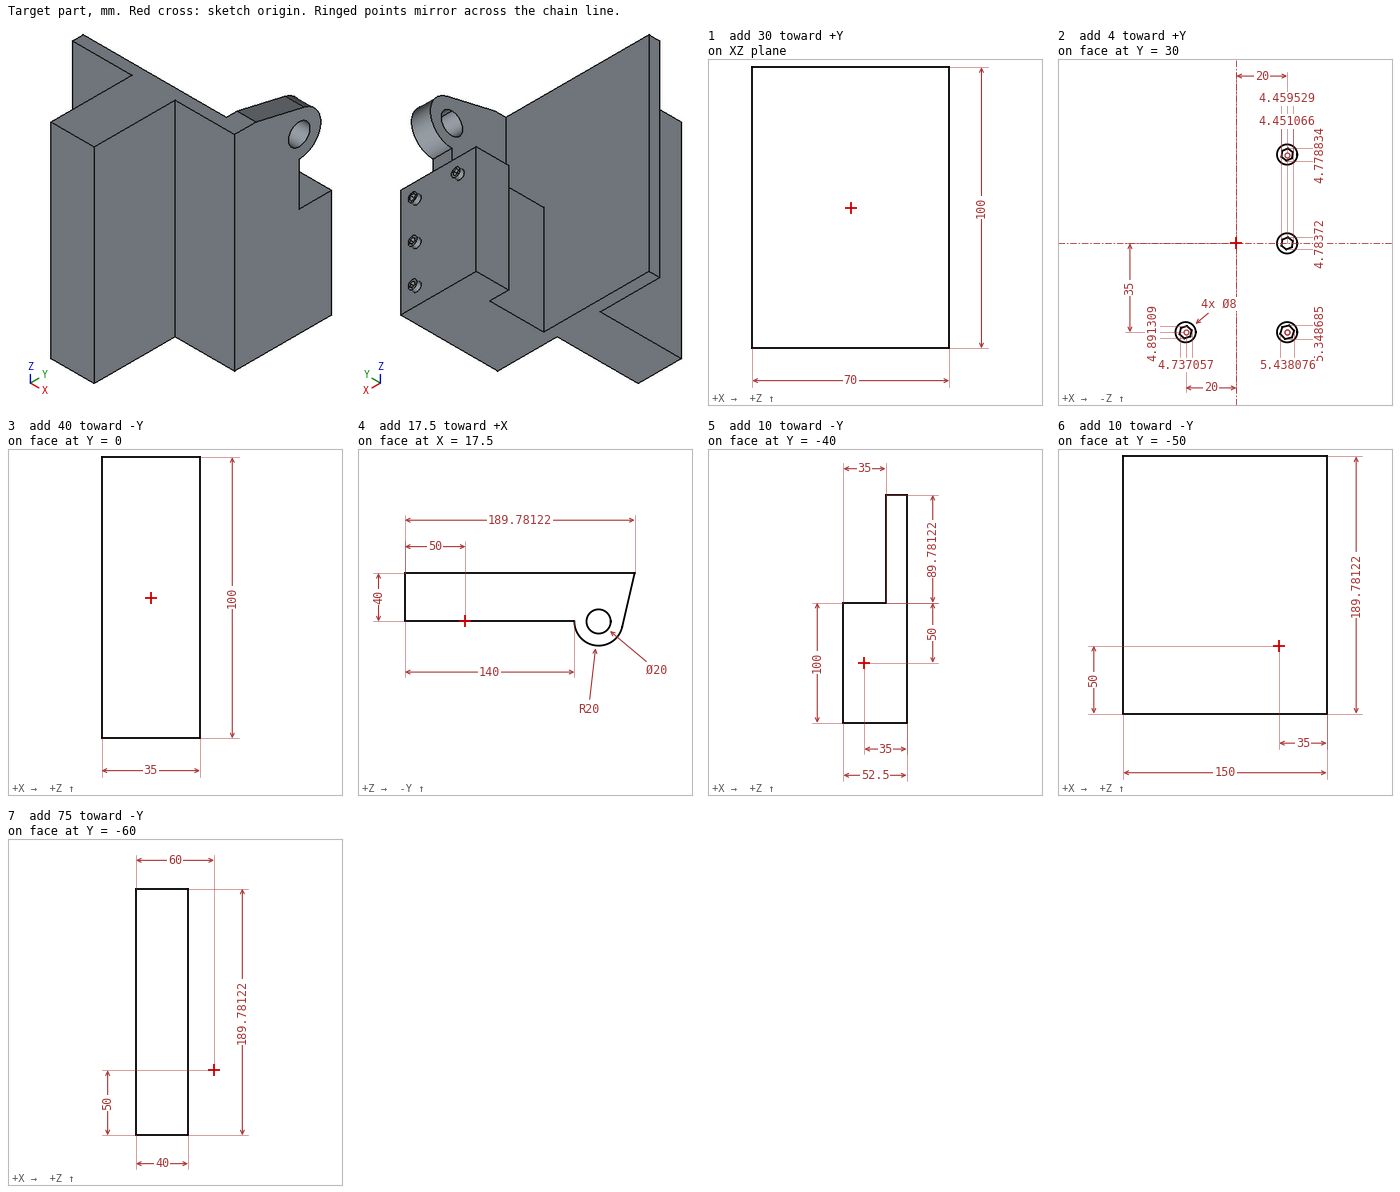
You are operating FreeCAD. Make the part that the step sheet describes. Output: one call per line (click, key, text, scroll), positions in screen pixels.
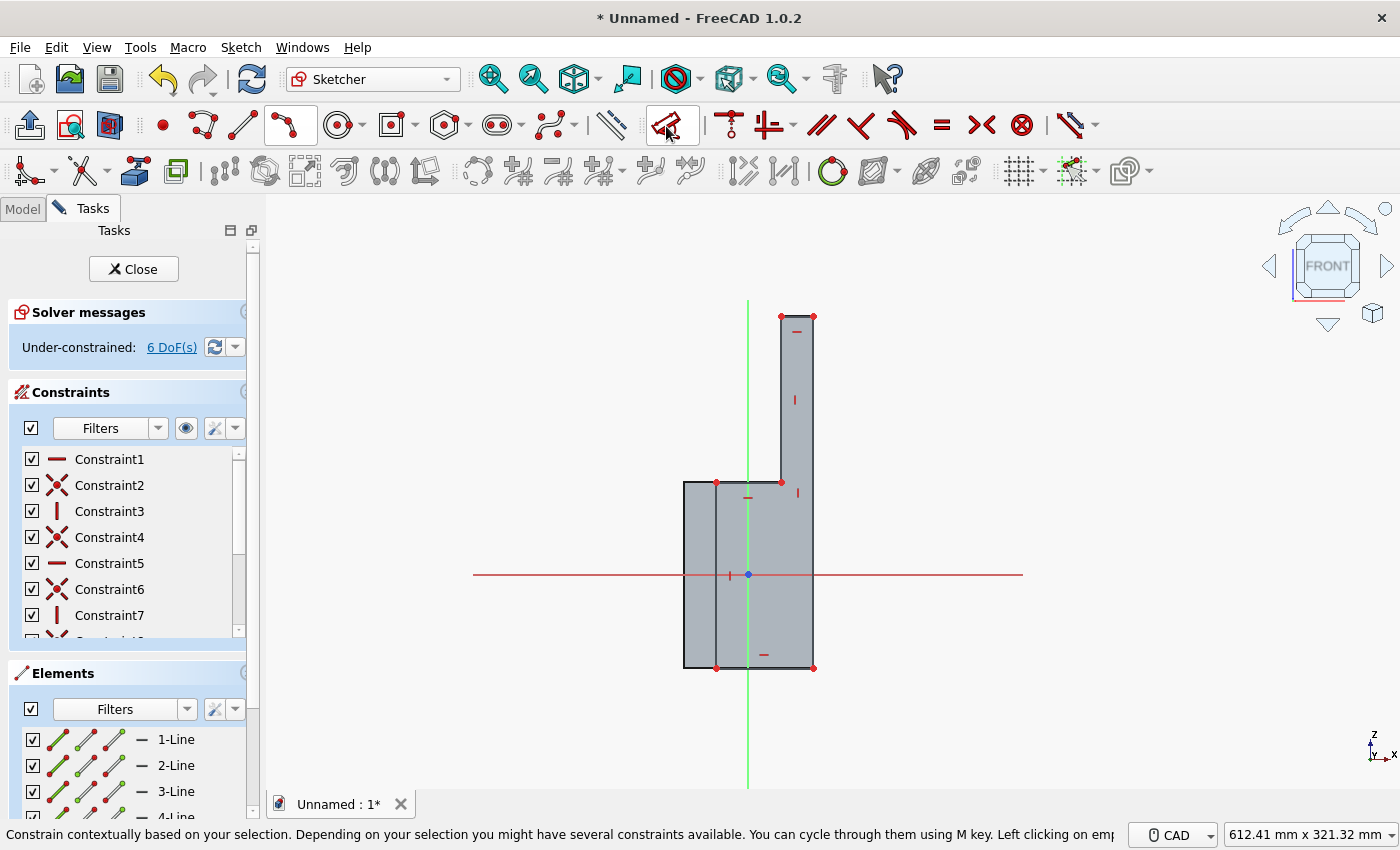
click(762, 483)
click(734, 449)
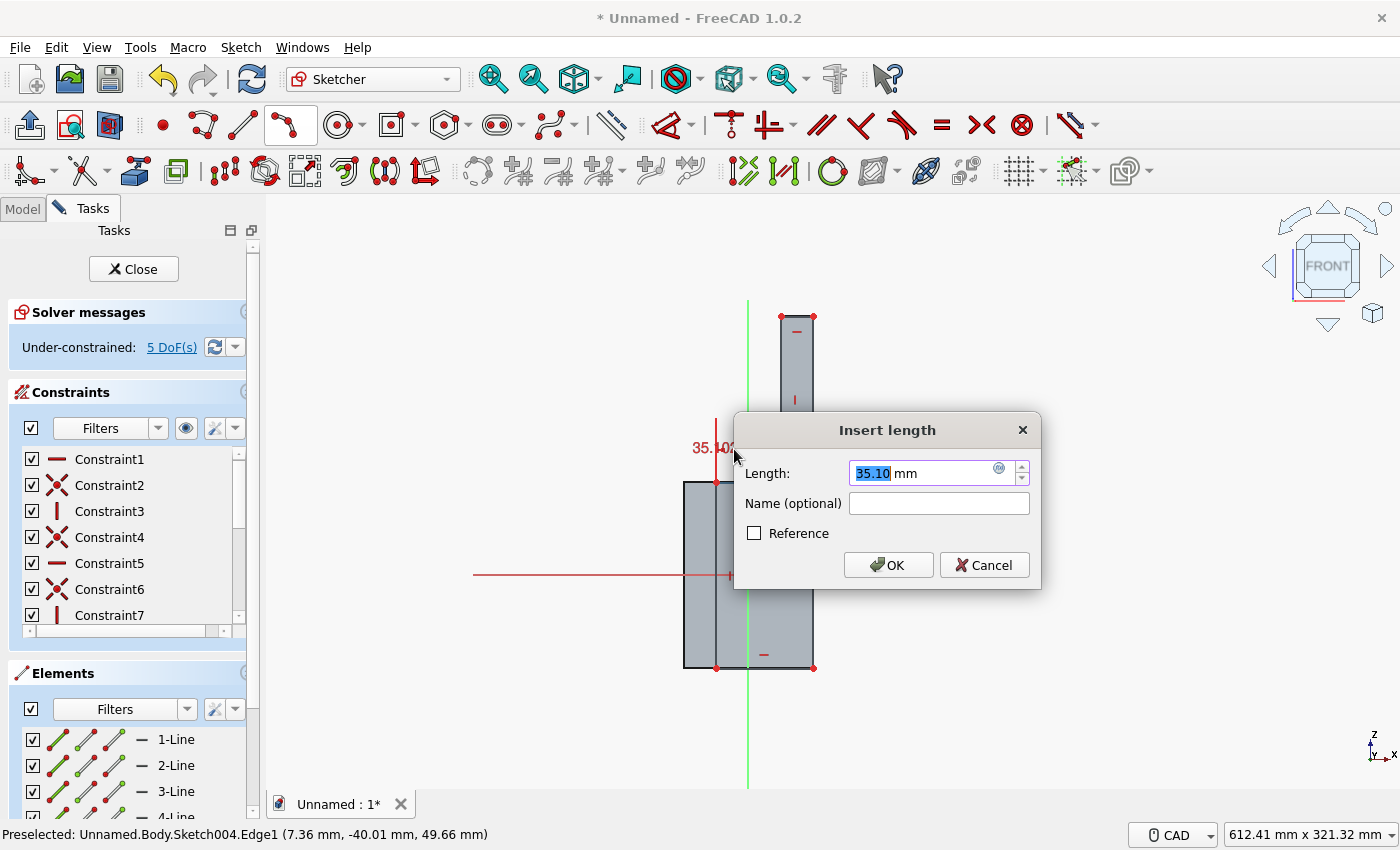
text(35)
key(Return)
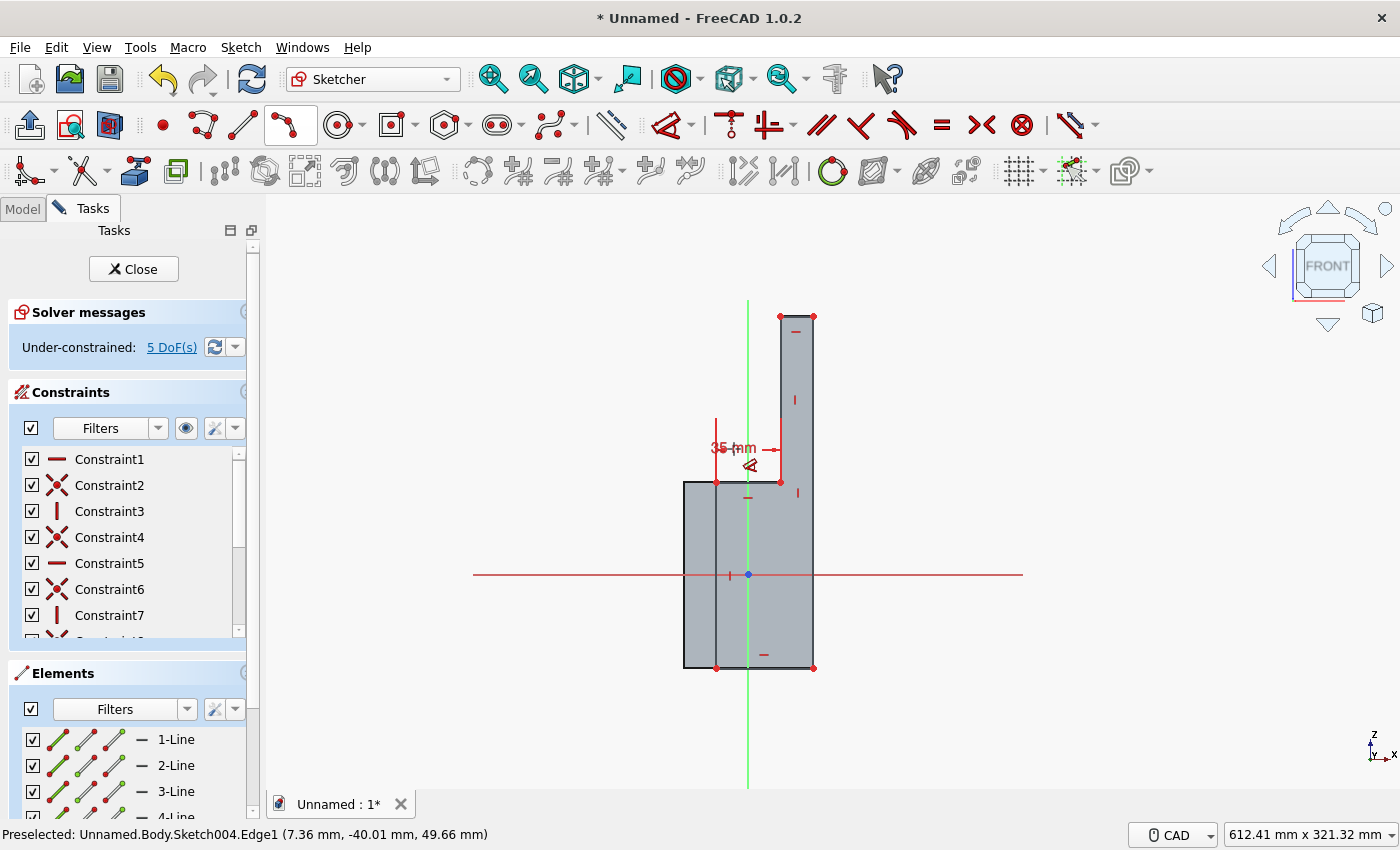
click(716, 539)
click(682, 533)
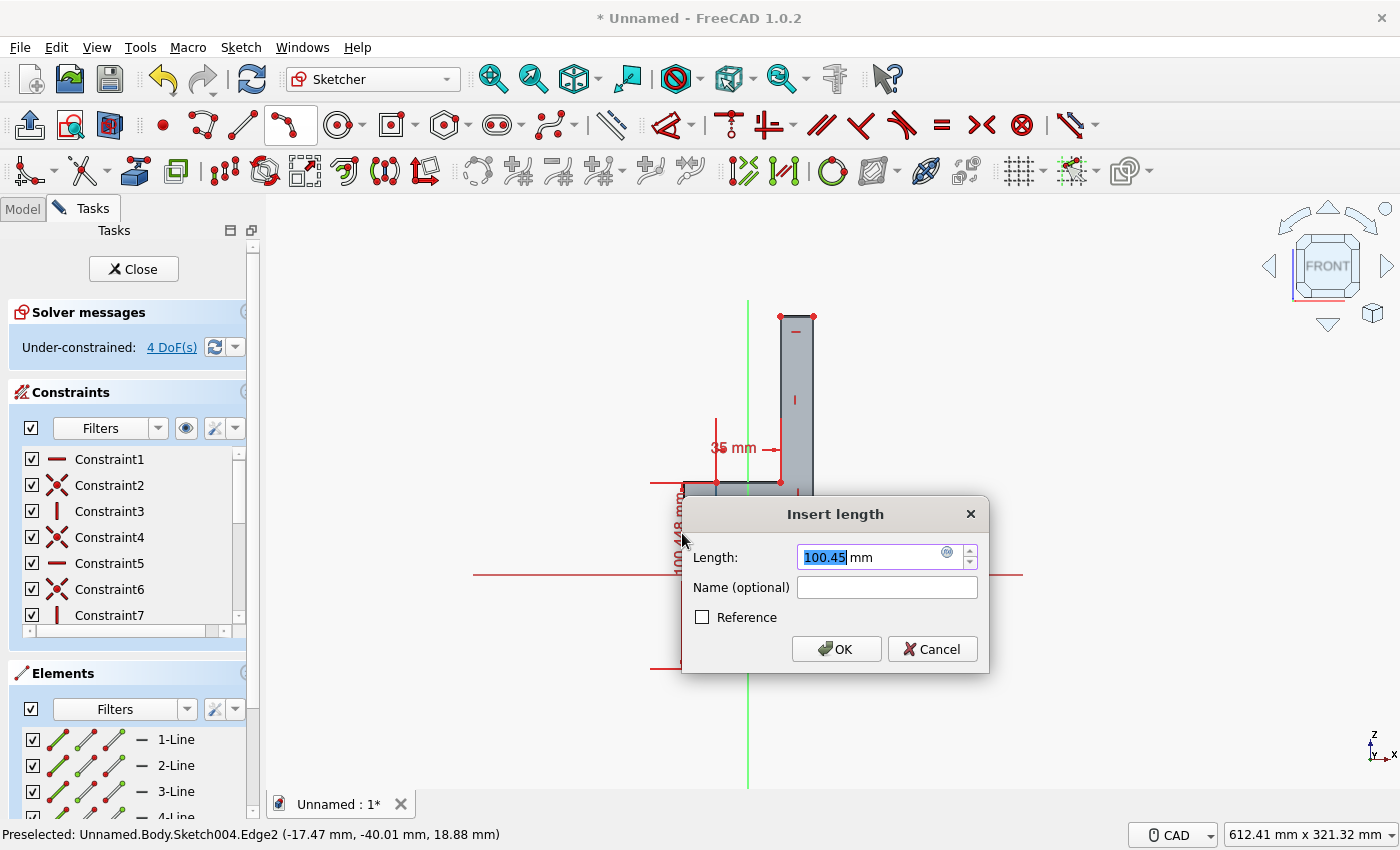
text(100)
key(Return)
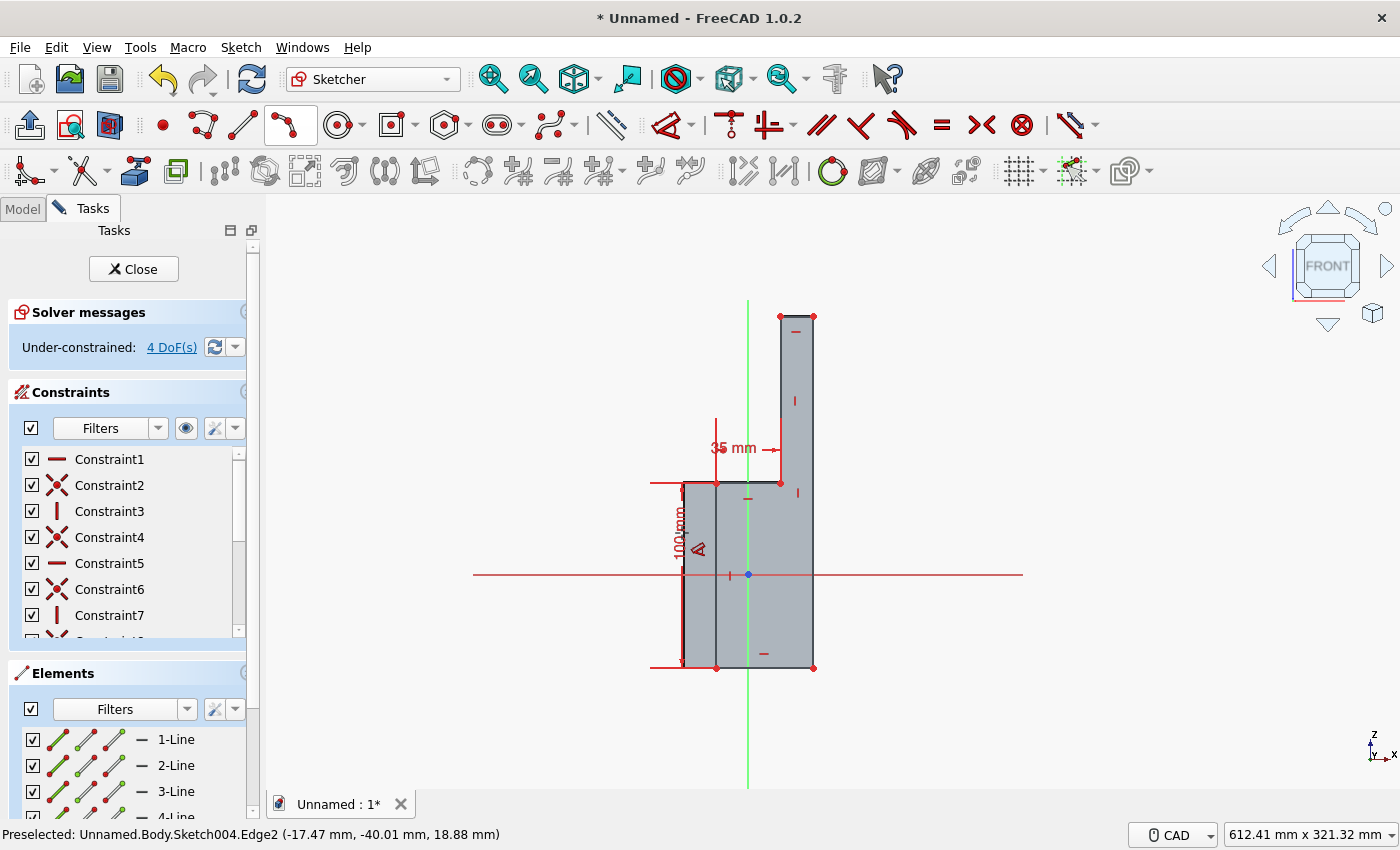
click(781, 483)
click(839, 529)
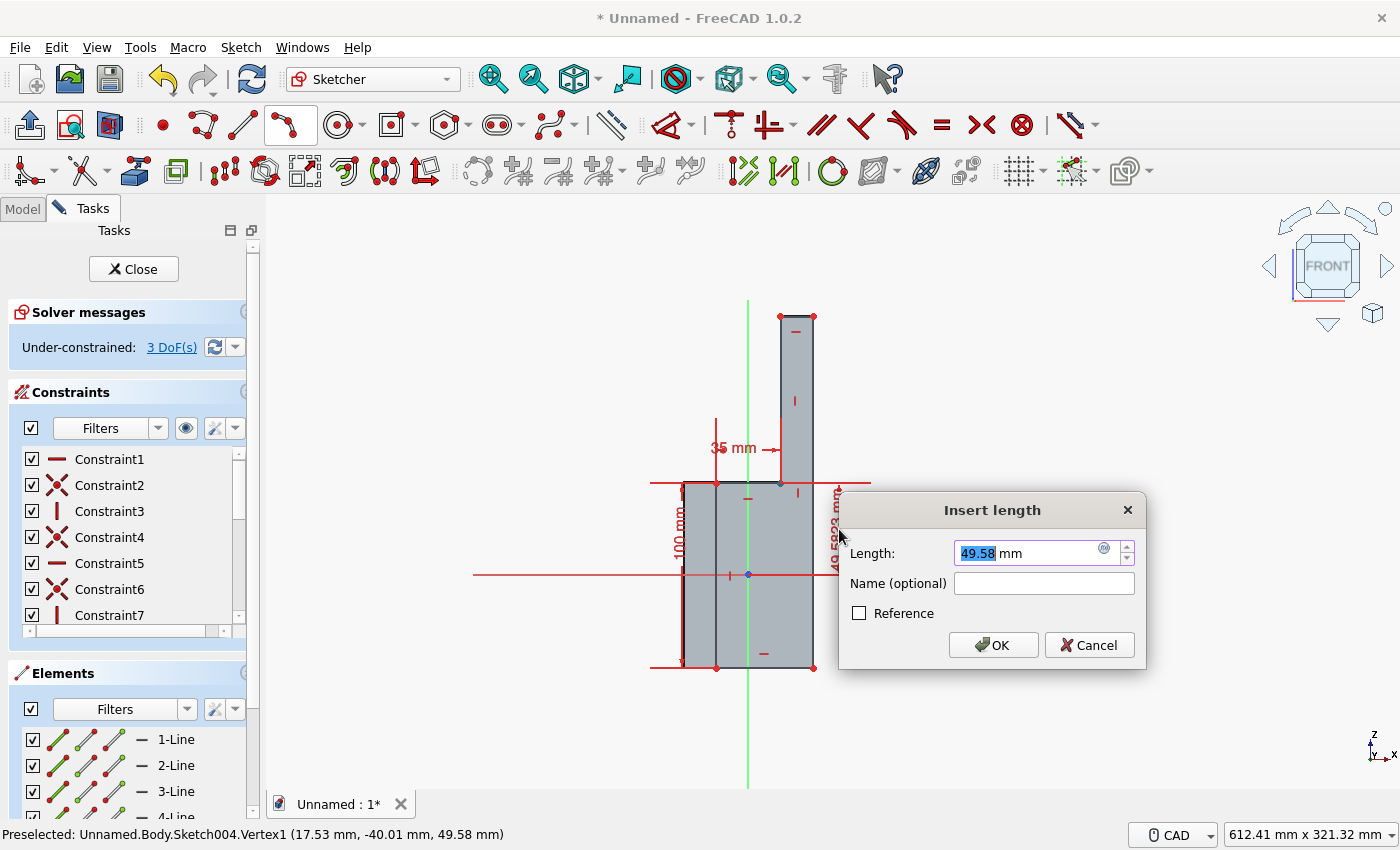
text(50)
key(Return)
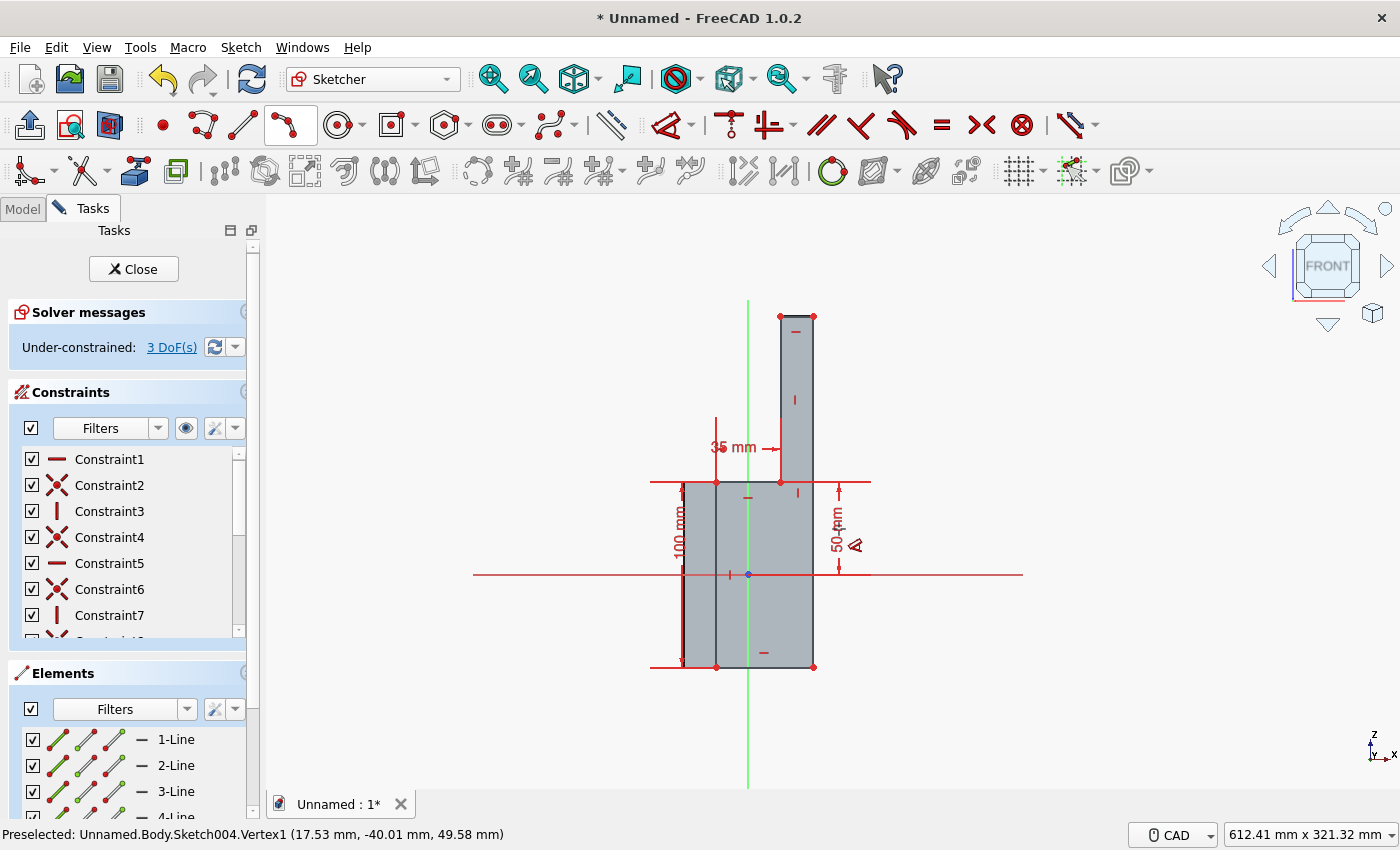
click(813, 668)
click(781, 702)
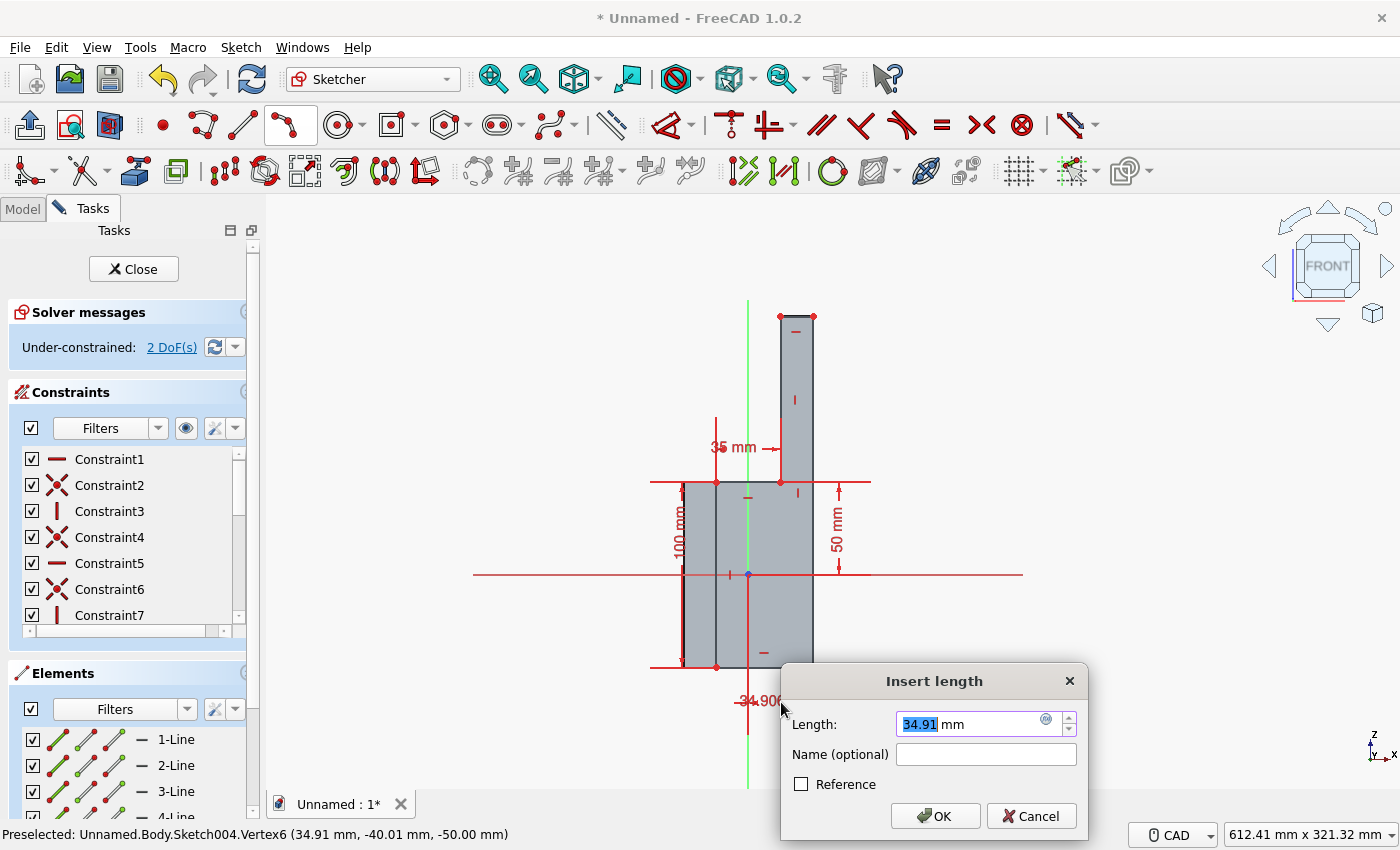
text(35)
key(Return)